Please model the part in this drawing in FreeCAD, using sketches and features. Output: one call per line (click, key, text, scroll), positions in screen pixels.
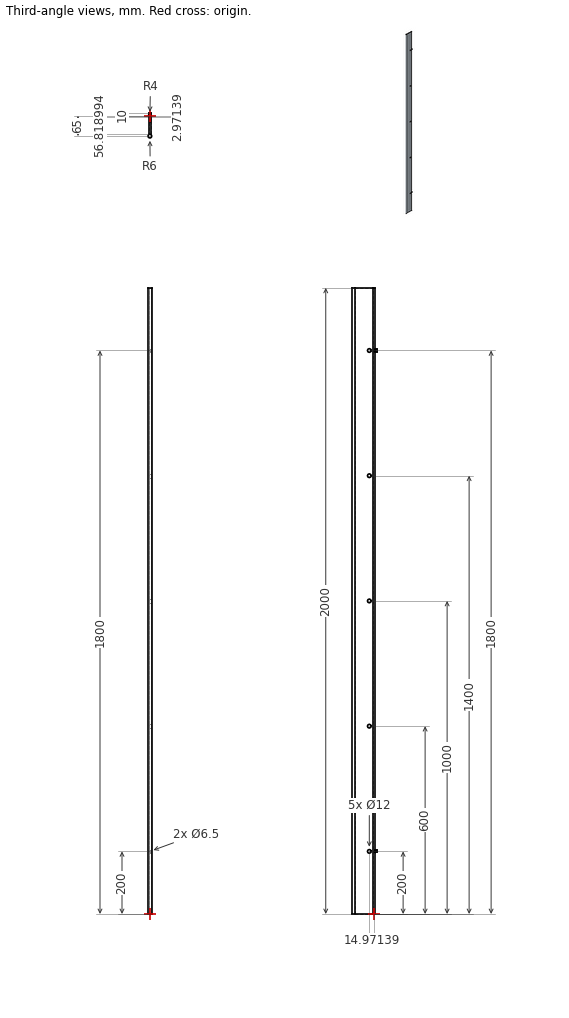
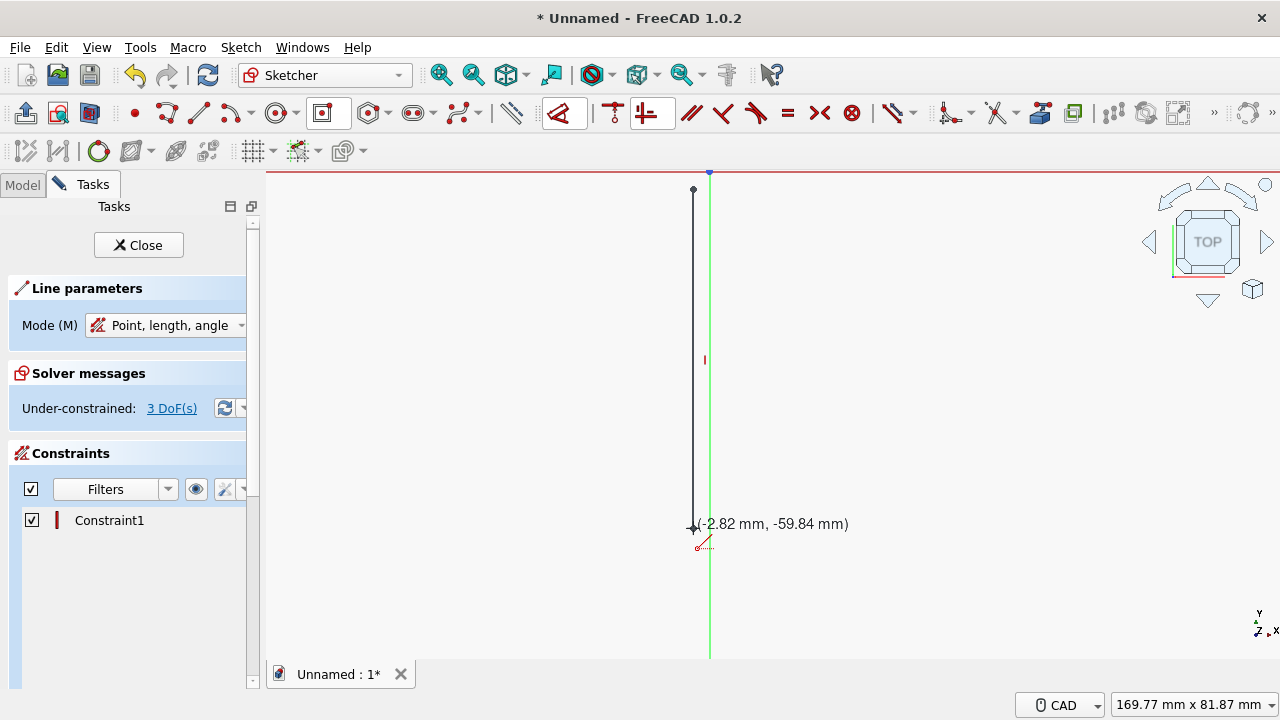
click(726, 528)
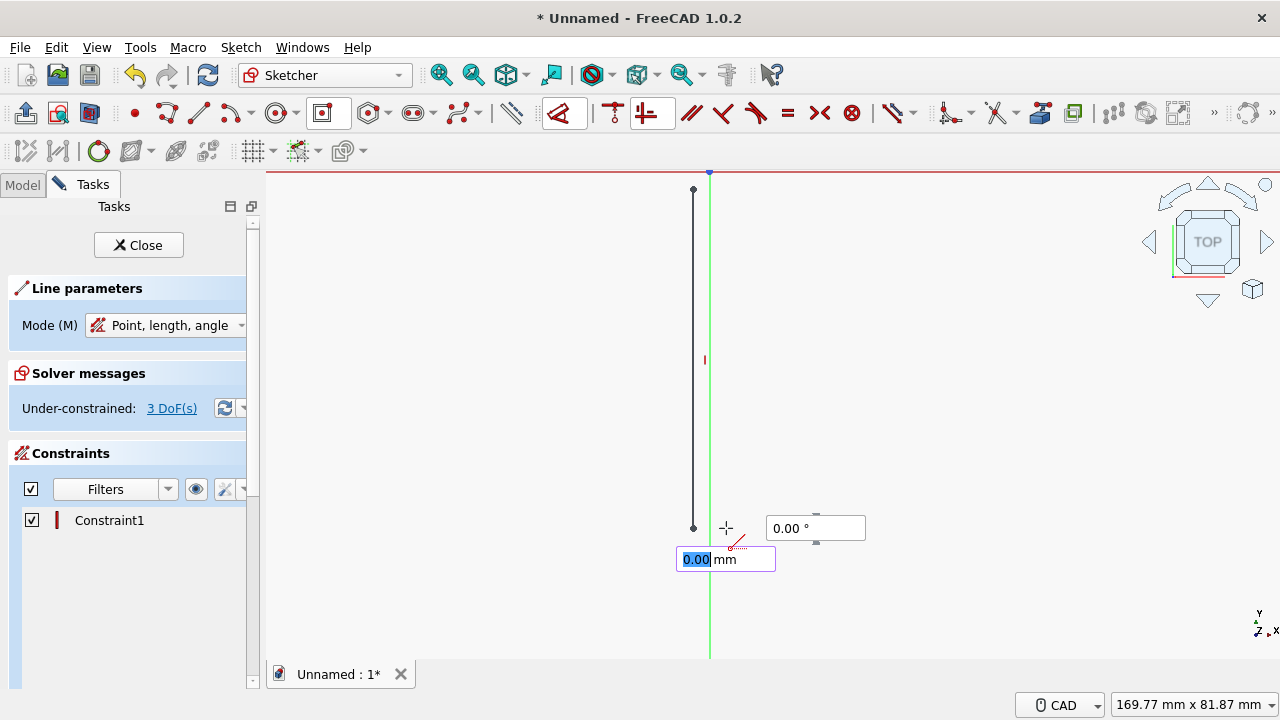
scroll(694, 502, down, 2)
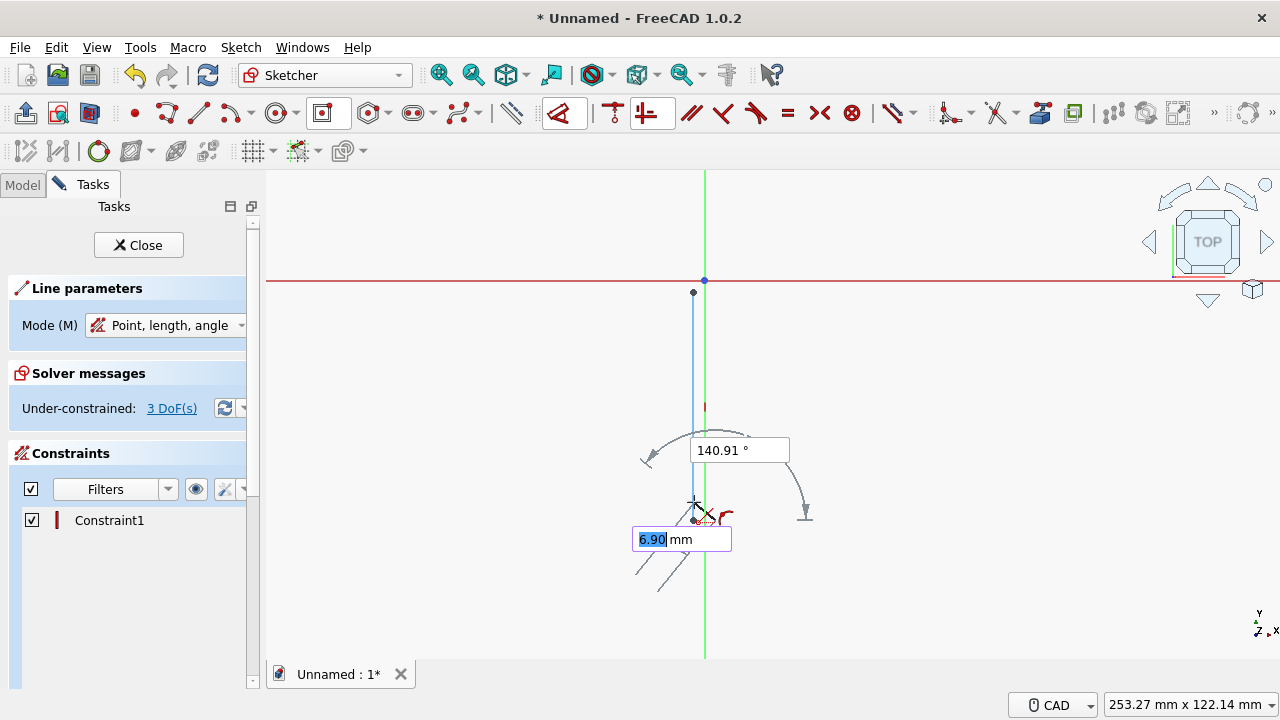
scroll(715, 293, up, 2)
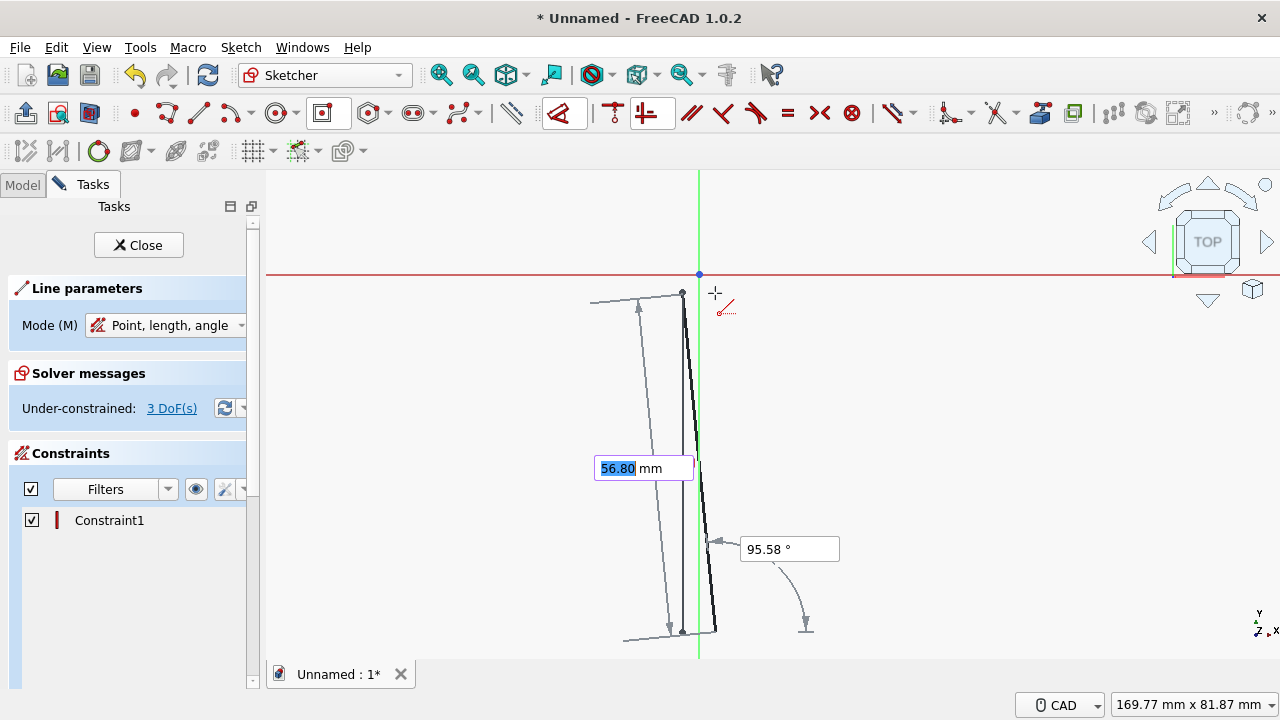
click(716, 292)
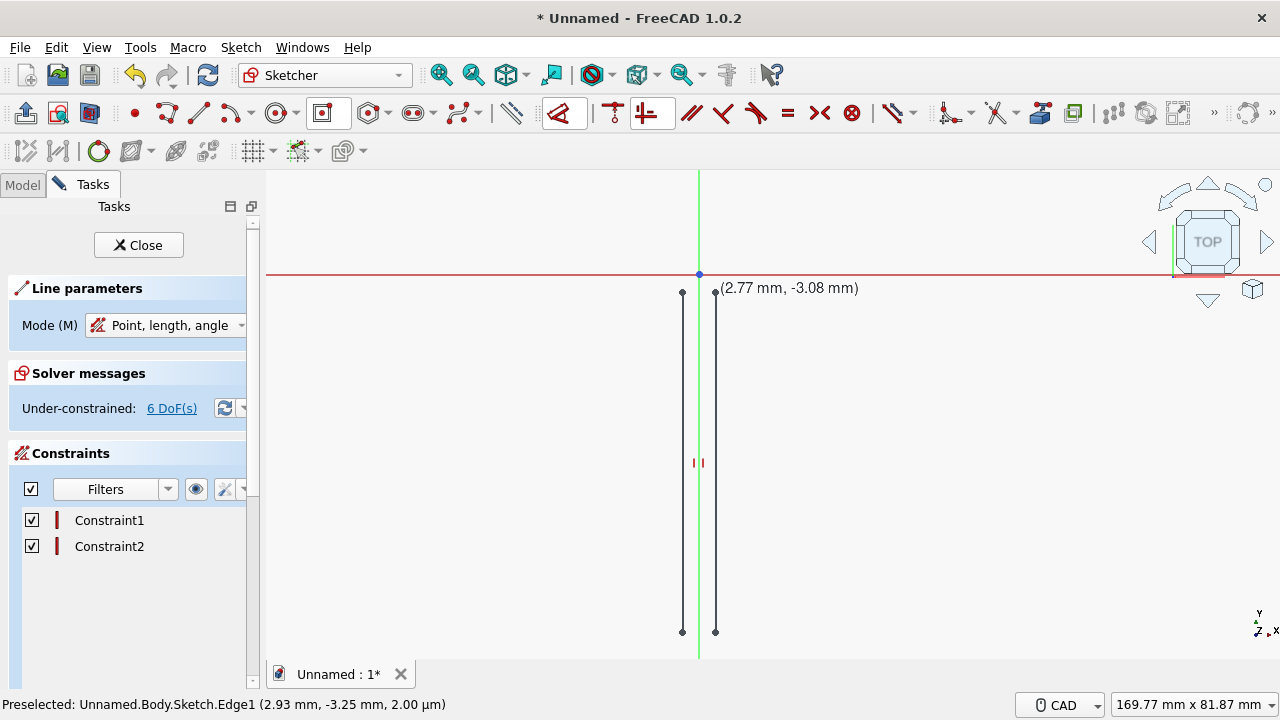
key(g)
key(3)
key(a)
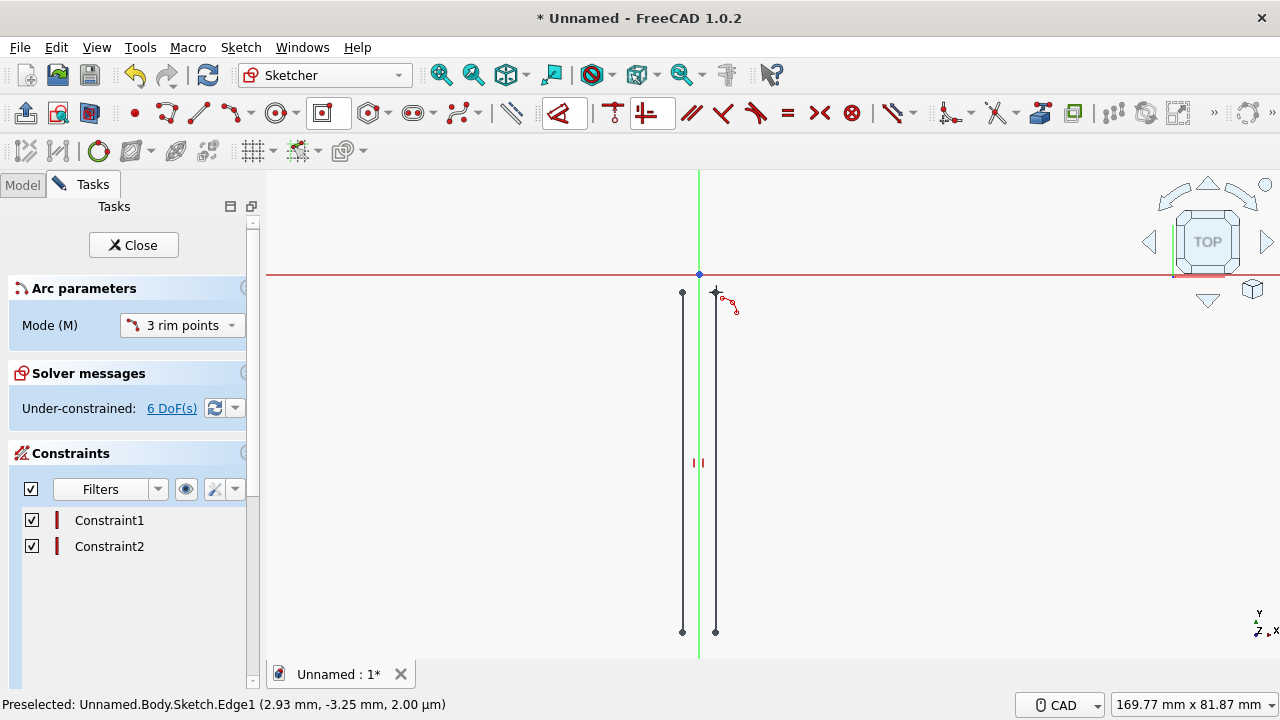
scroll(715, 292, down, 2)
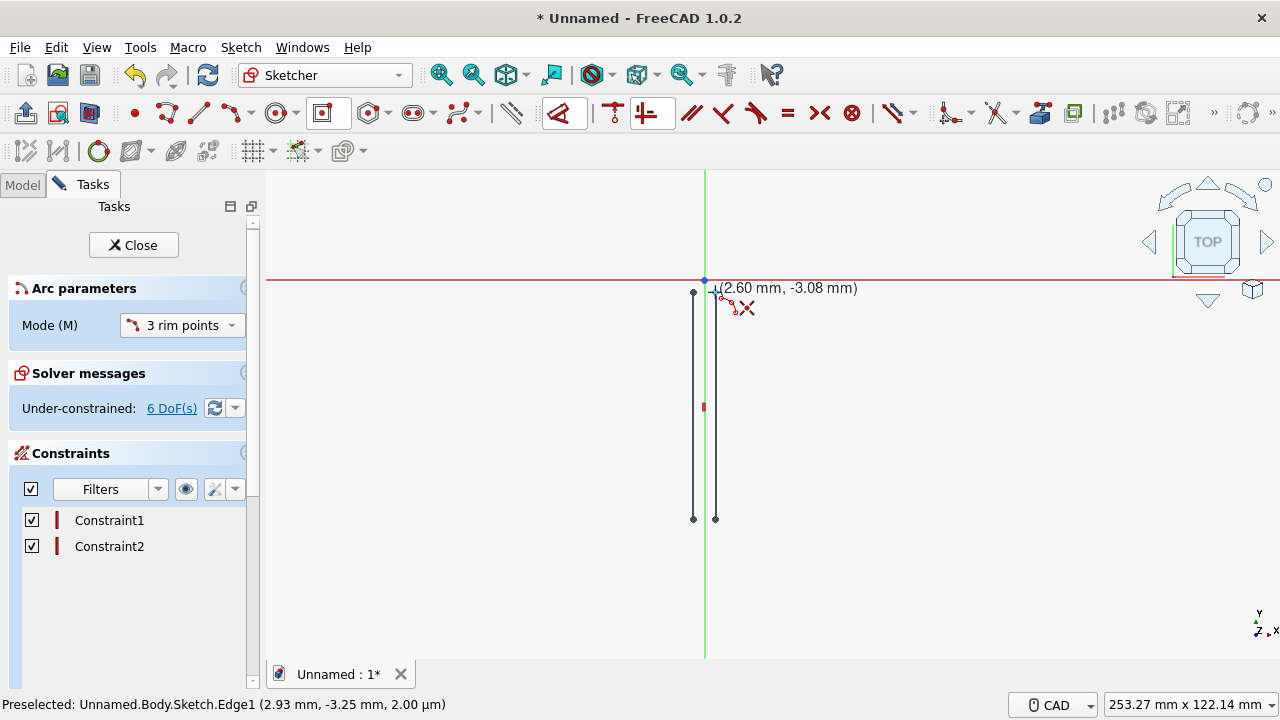
scroll(694, 519, up, 2)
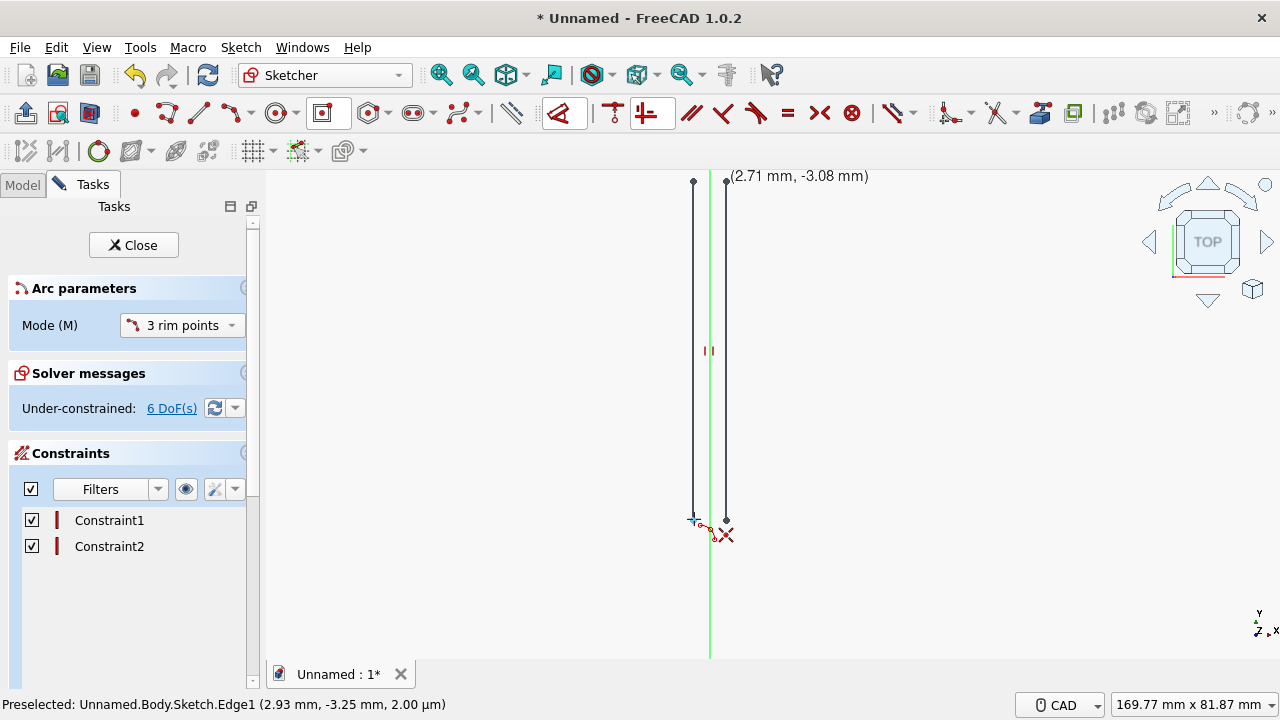
click(693, 520)
click(726, 520)
click(679, 569)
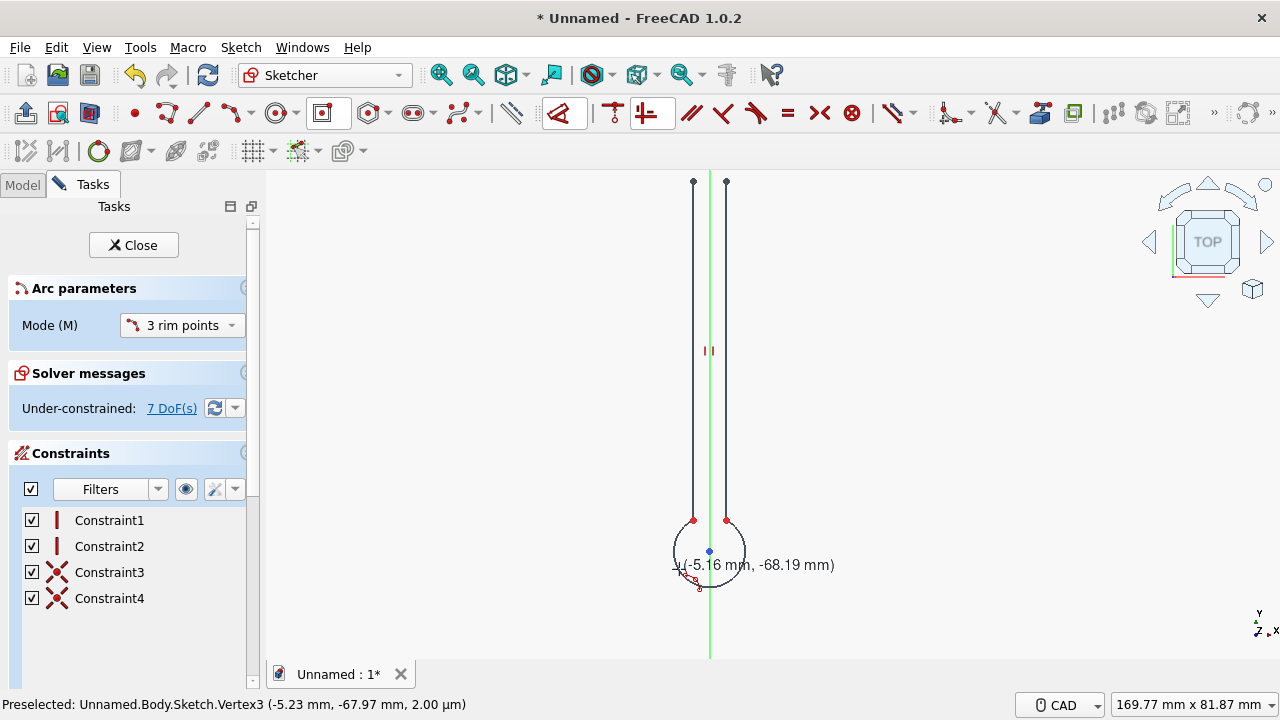
scroll(694, 520, down, 2)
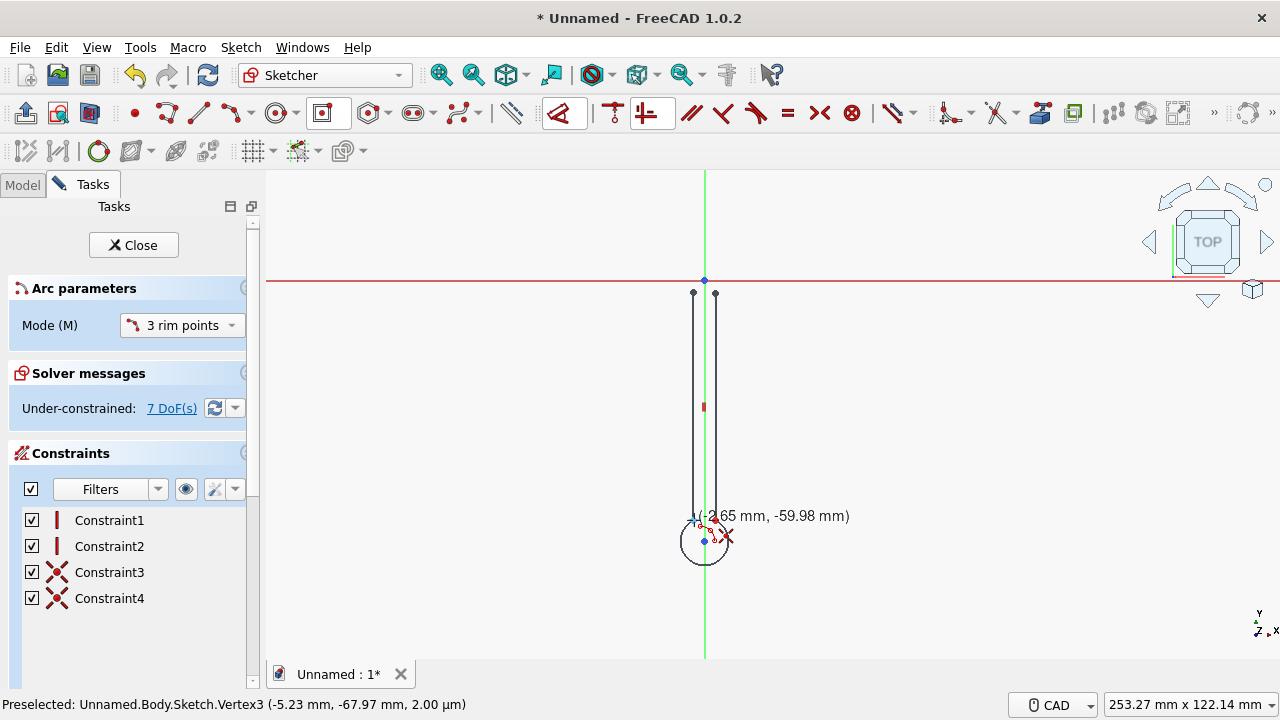
scroll(715, 293, up, 2)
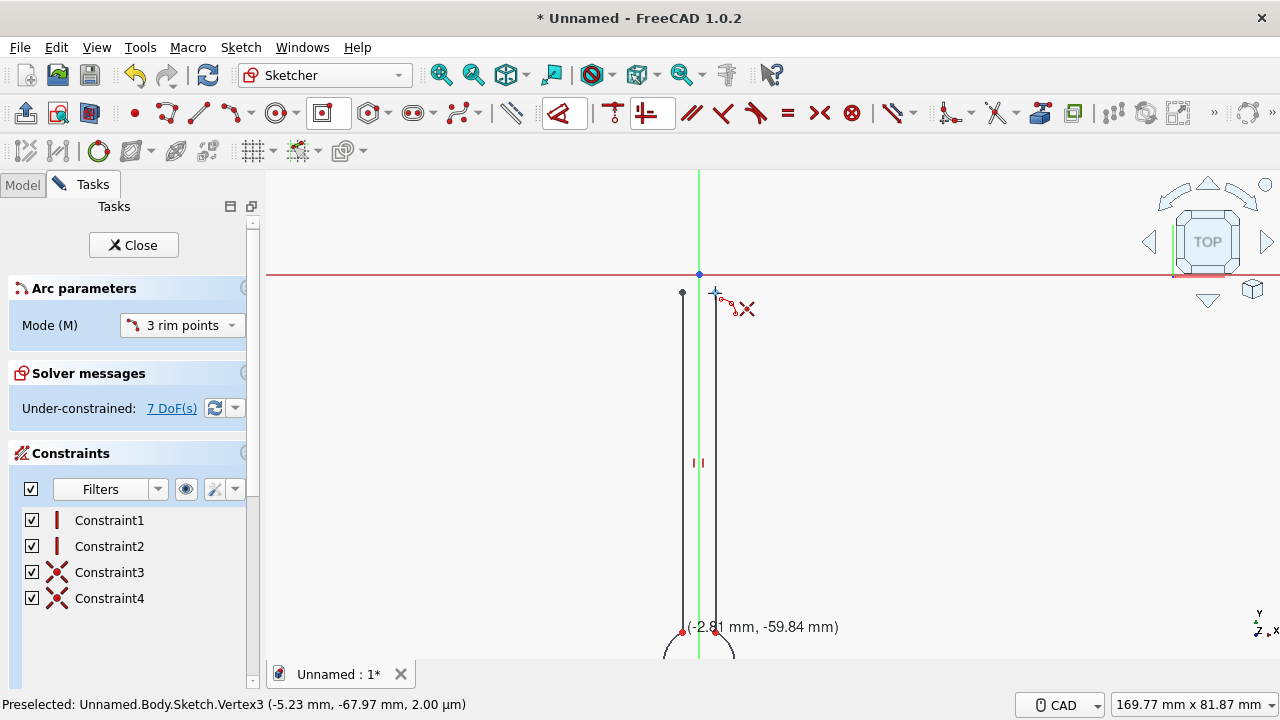
click(716, 293)
click(683, 293)
click(680, 260)
key(Escape)